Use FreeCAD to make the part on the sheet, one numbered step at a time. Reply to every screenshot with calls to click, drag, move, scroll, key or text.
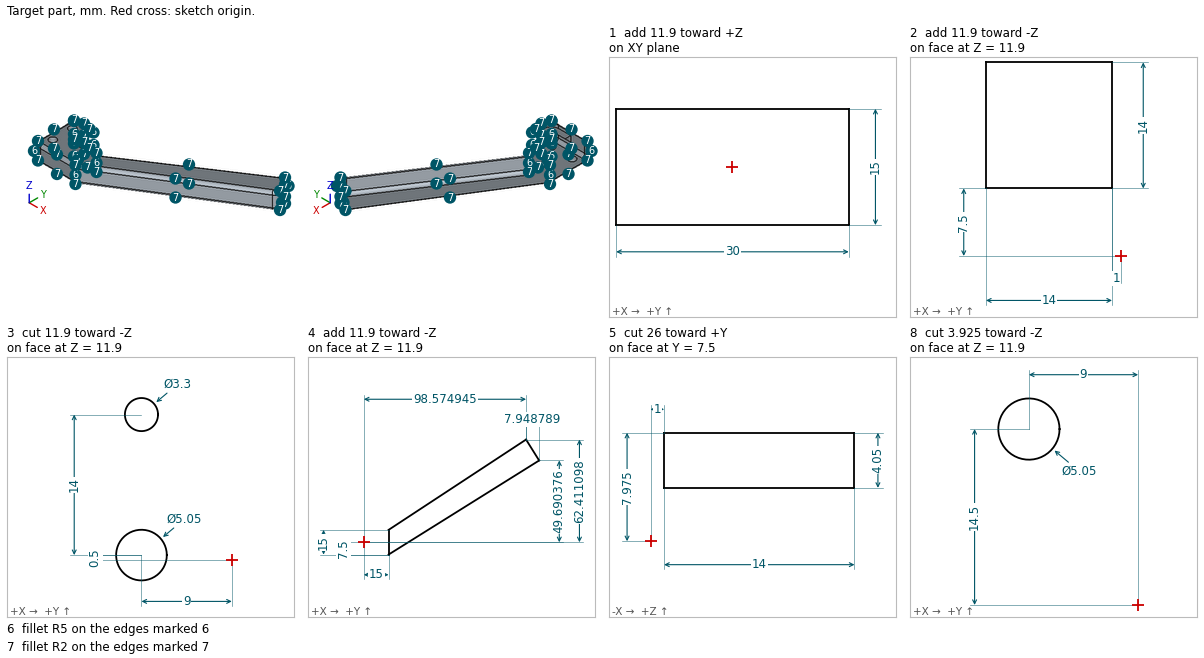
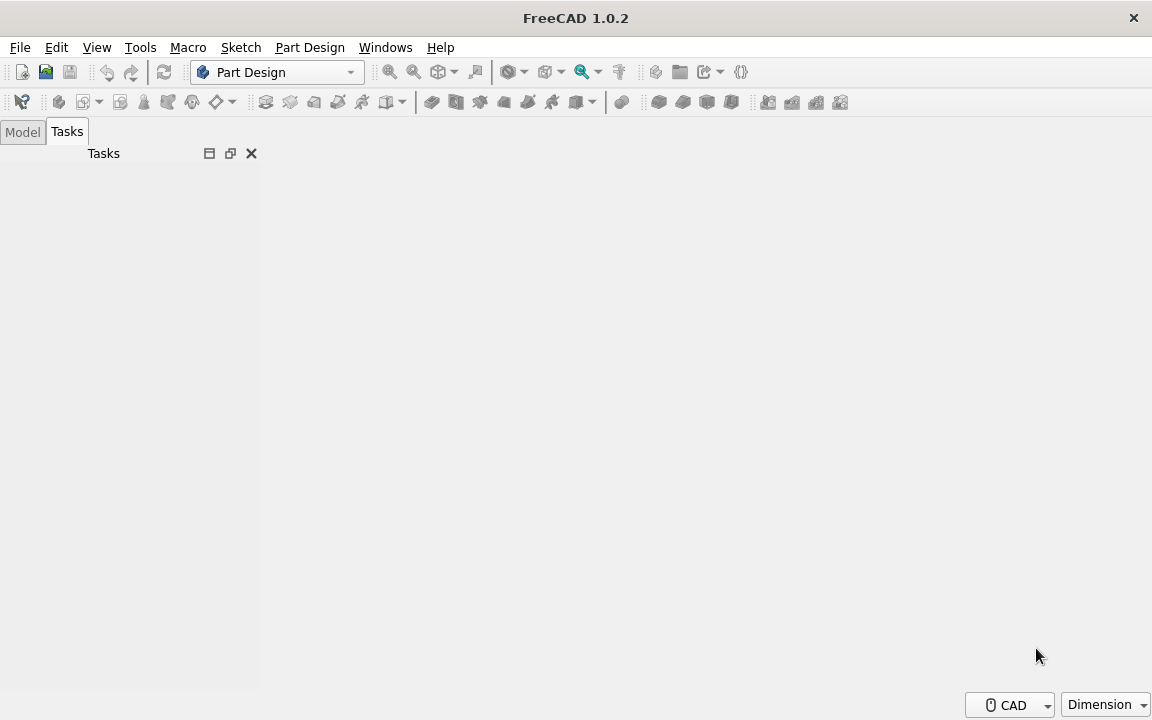
click(22, 72)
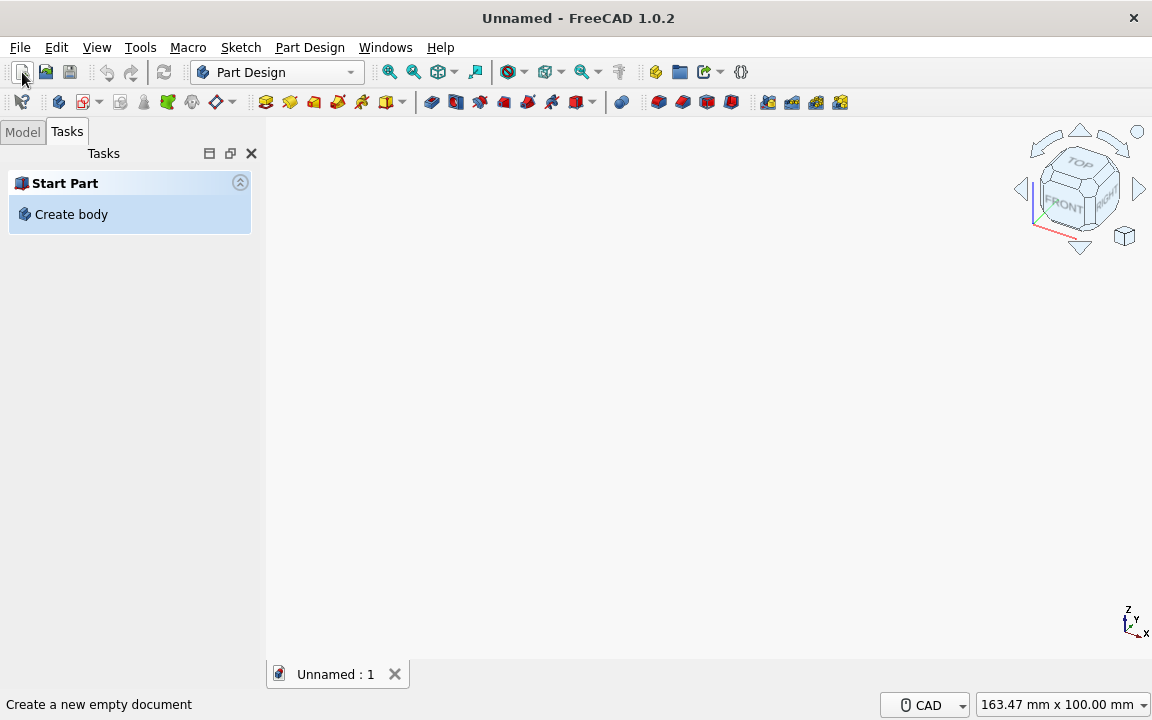
click(84, 102)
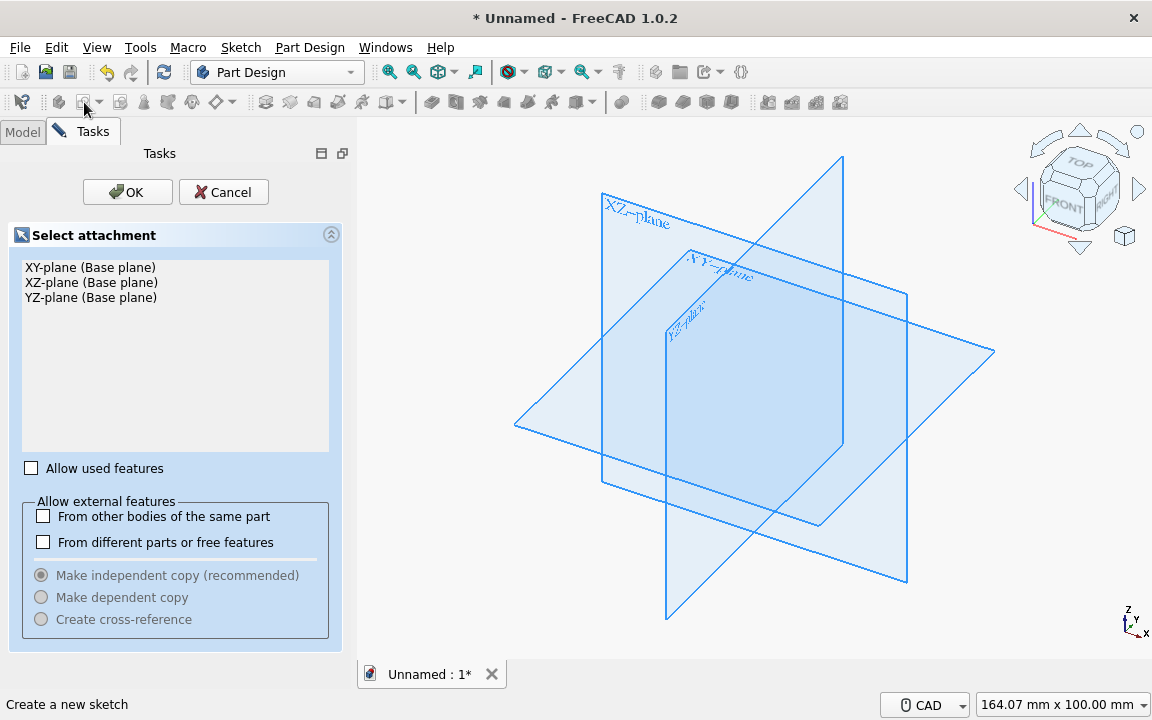
click(82, 268)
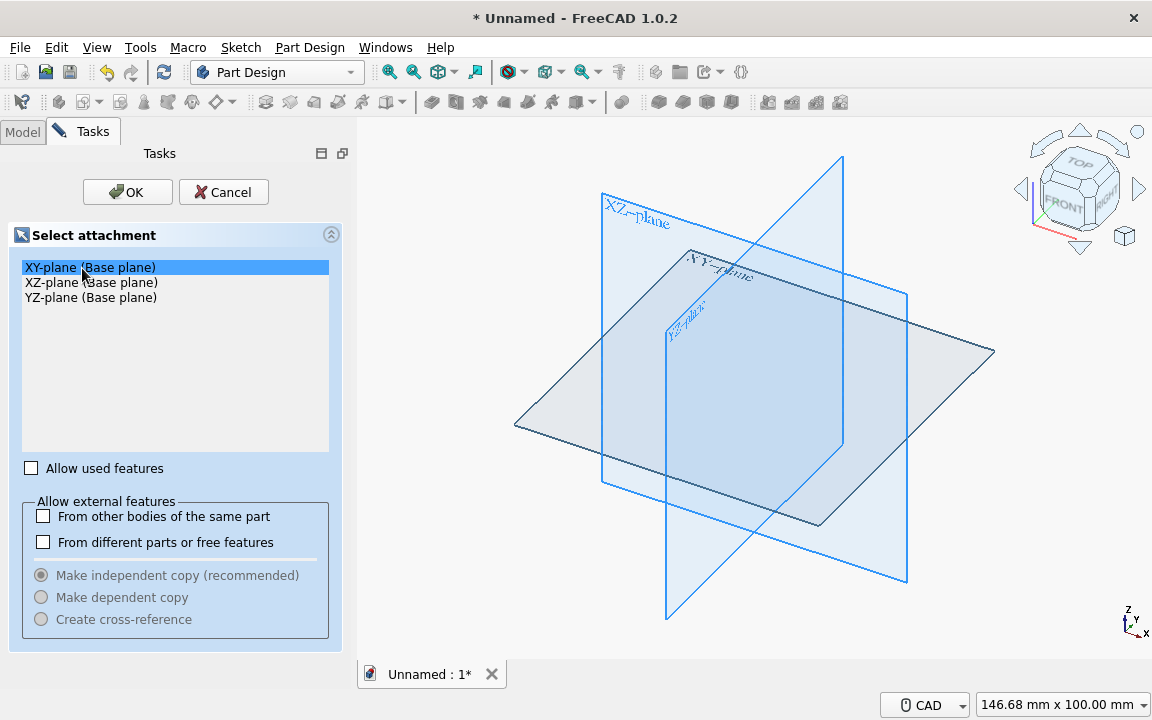
click(128, 192)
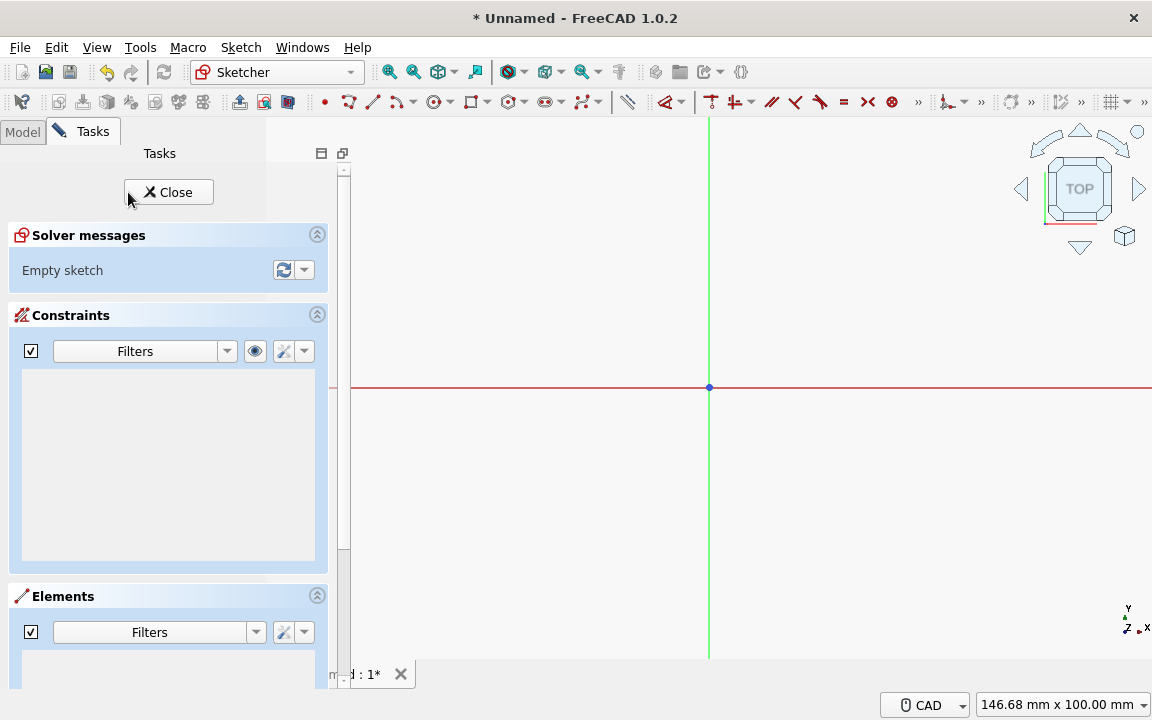
scroll(739, 388, up, 6)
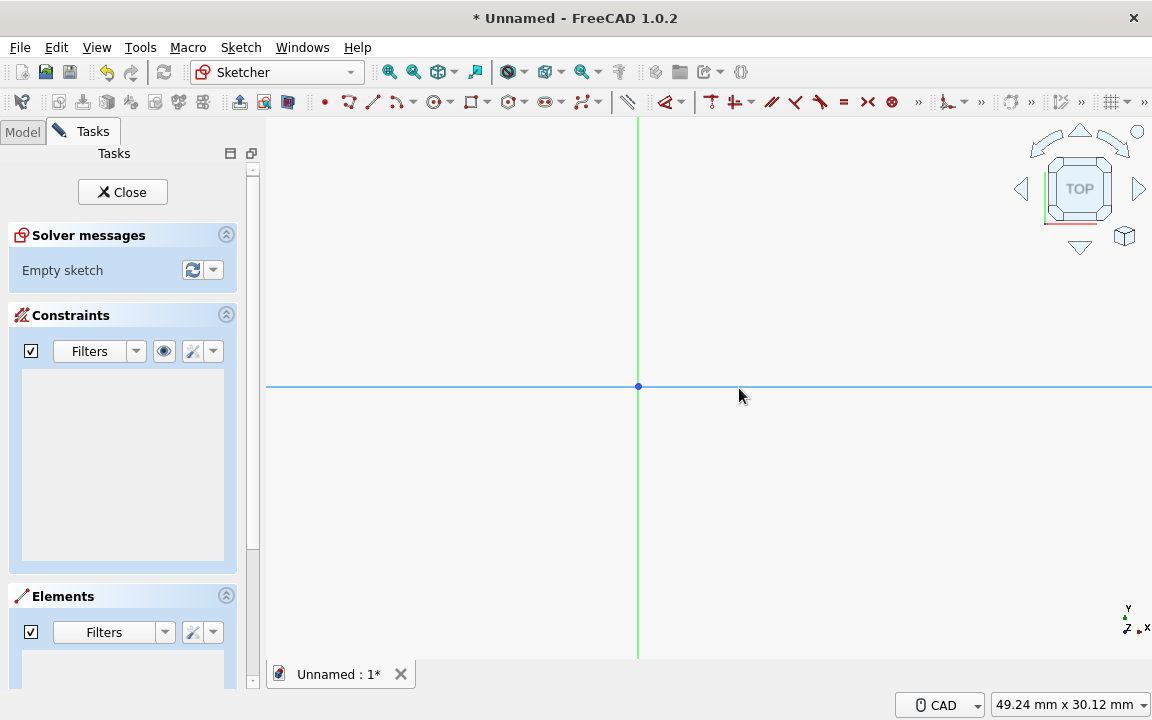
click(490, 102)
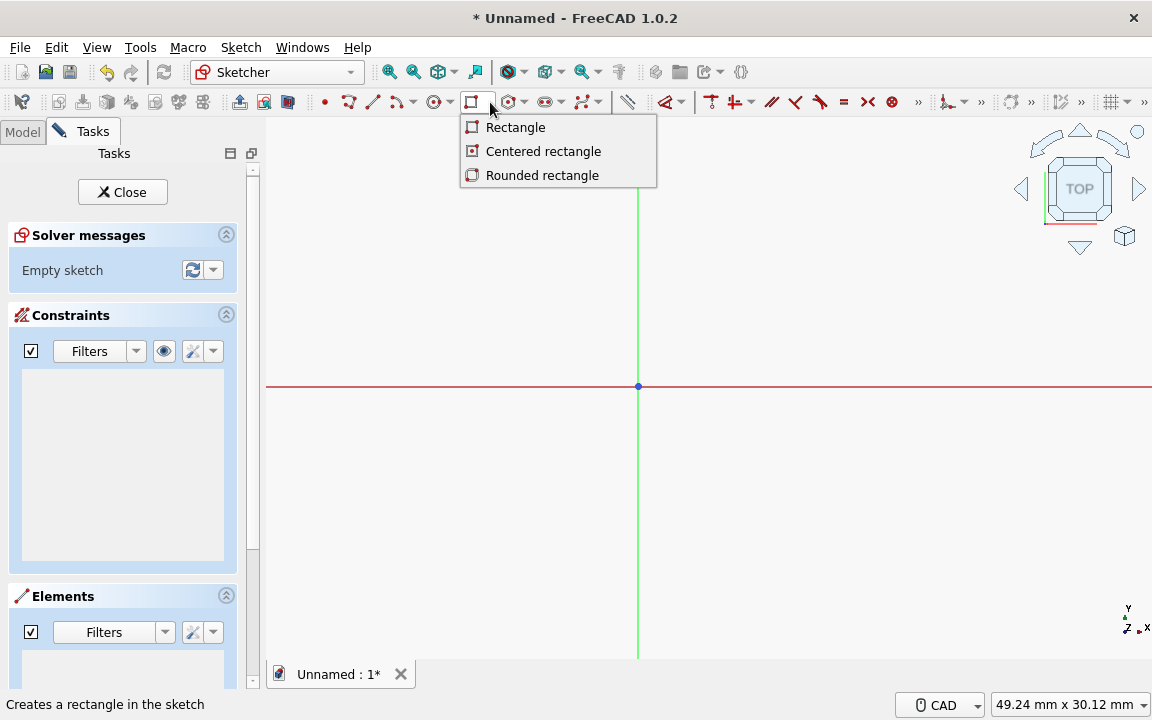
click(558, 151)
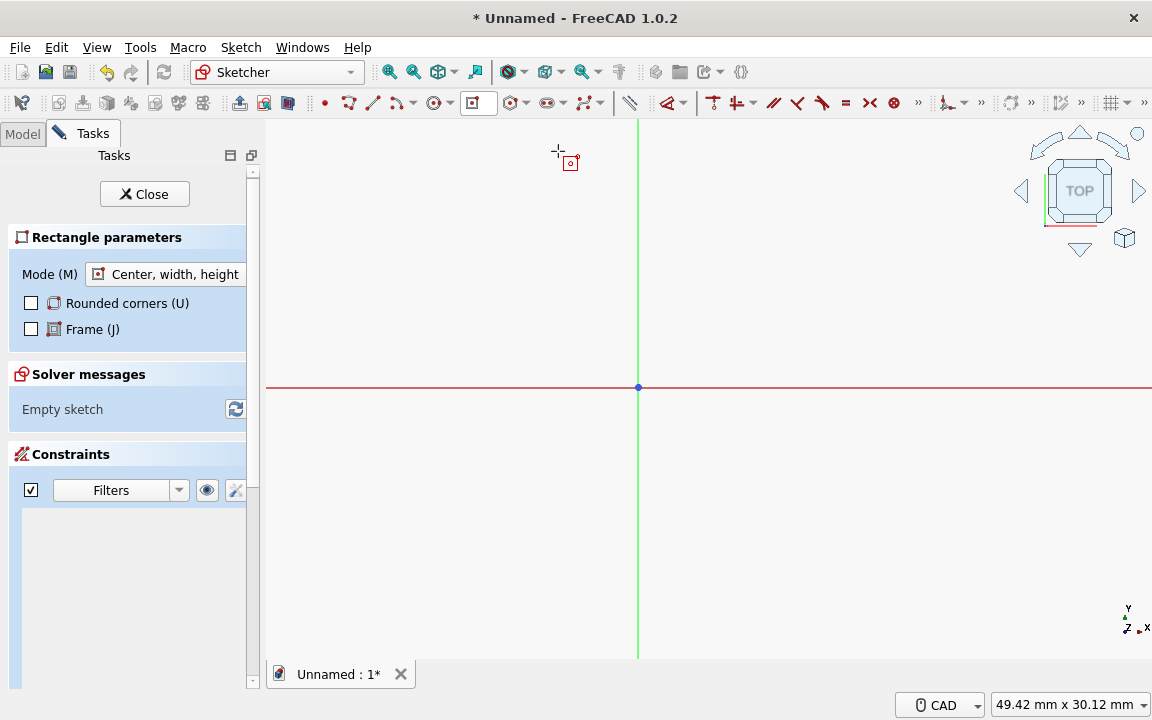
click(638, 388)
move(907, 253)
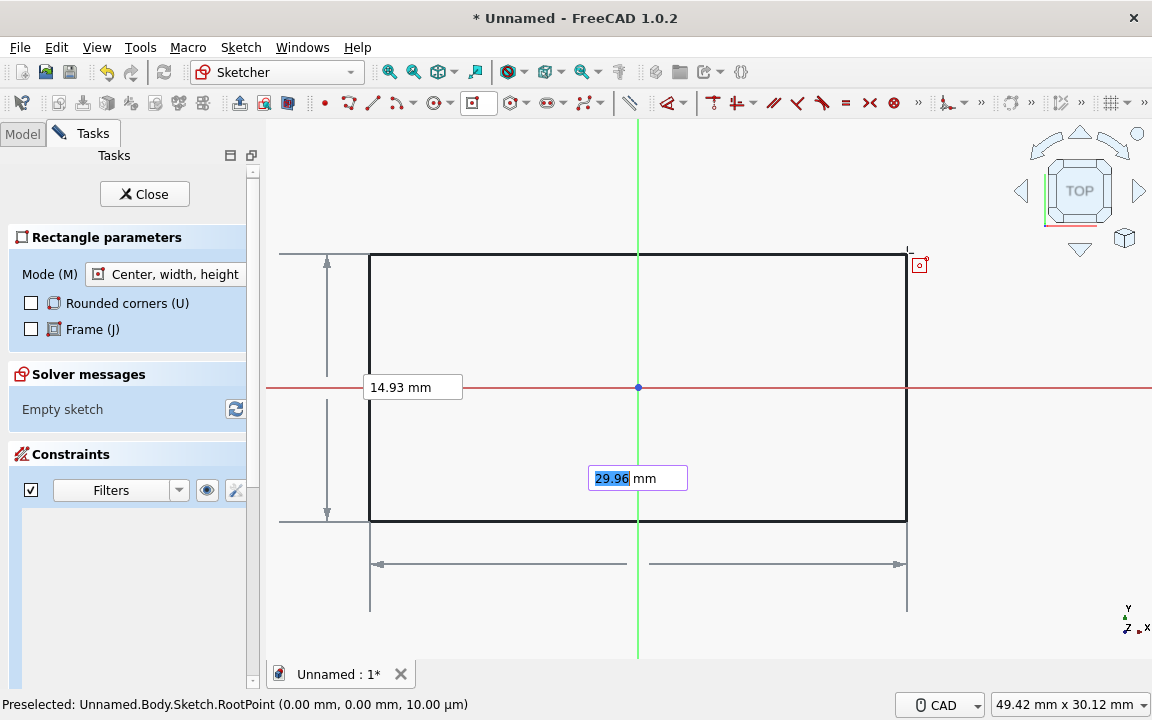
text(30)
key(Tab)
text(15)
key(Return)
key(Escape)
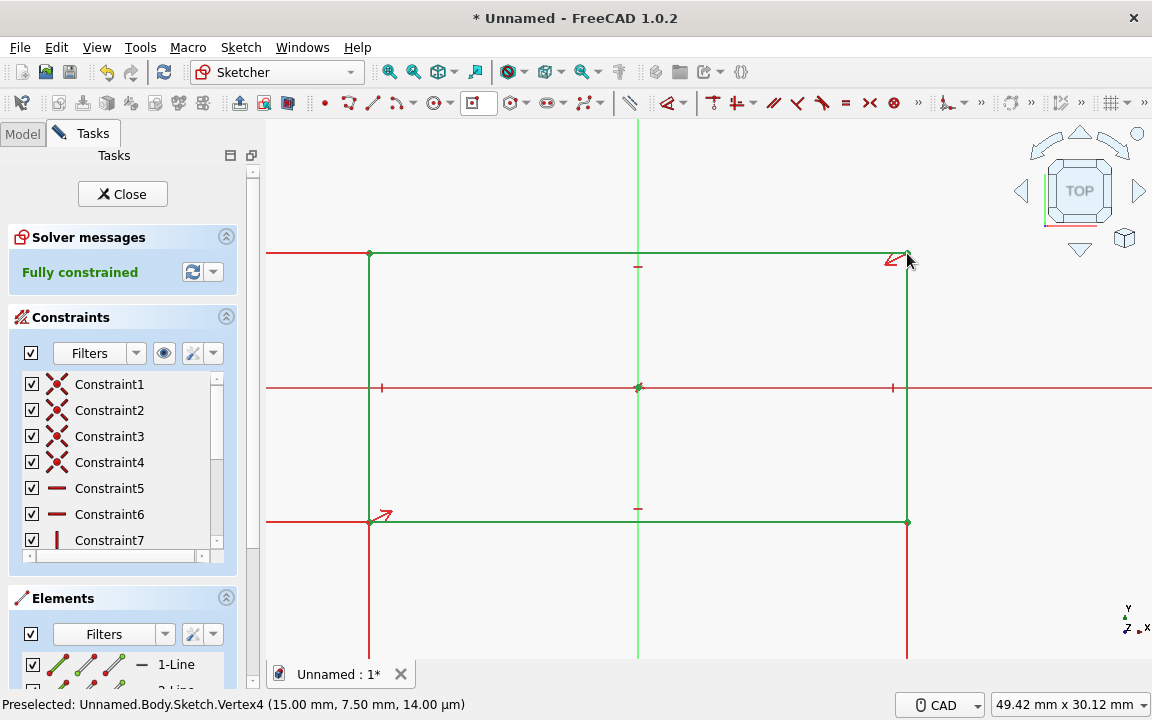
click(123, 194)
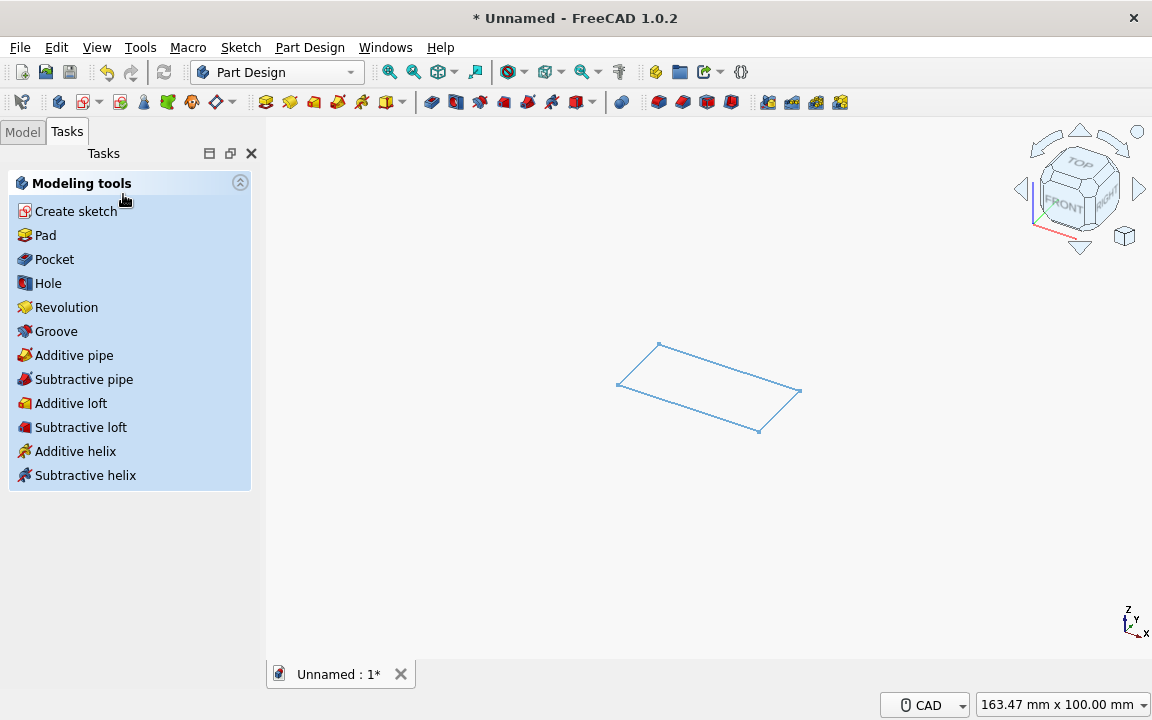
click(266, 102)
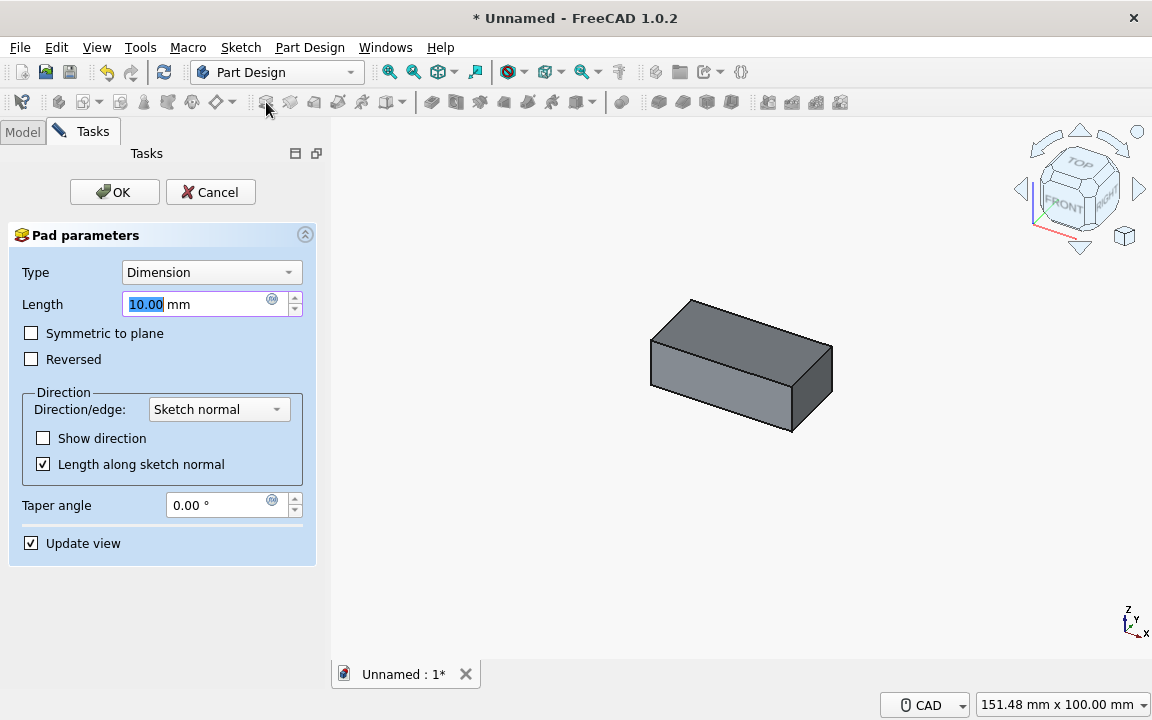
text(11.9)
key(Tab)